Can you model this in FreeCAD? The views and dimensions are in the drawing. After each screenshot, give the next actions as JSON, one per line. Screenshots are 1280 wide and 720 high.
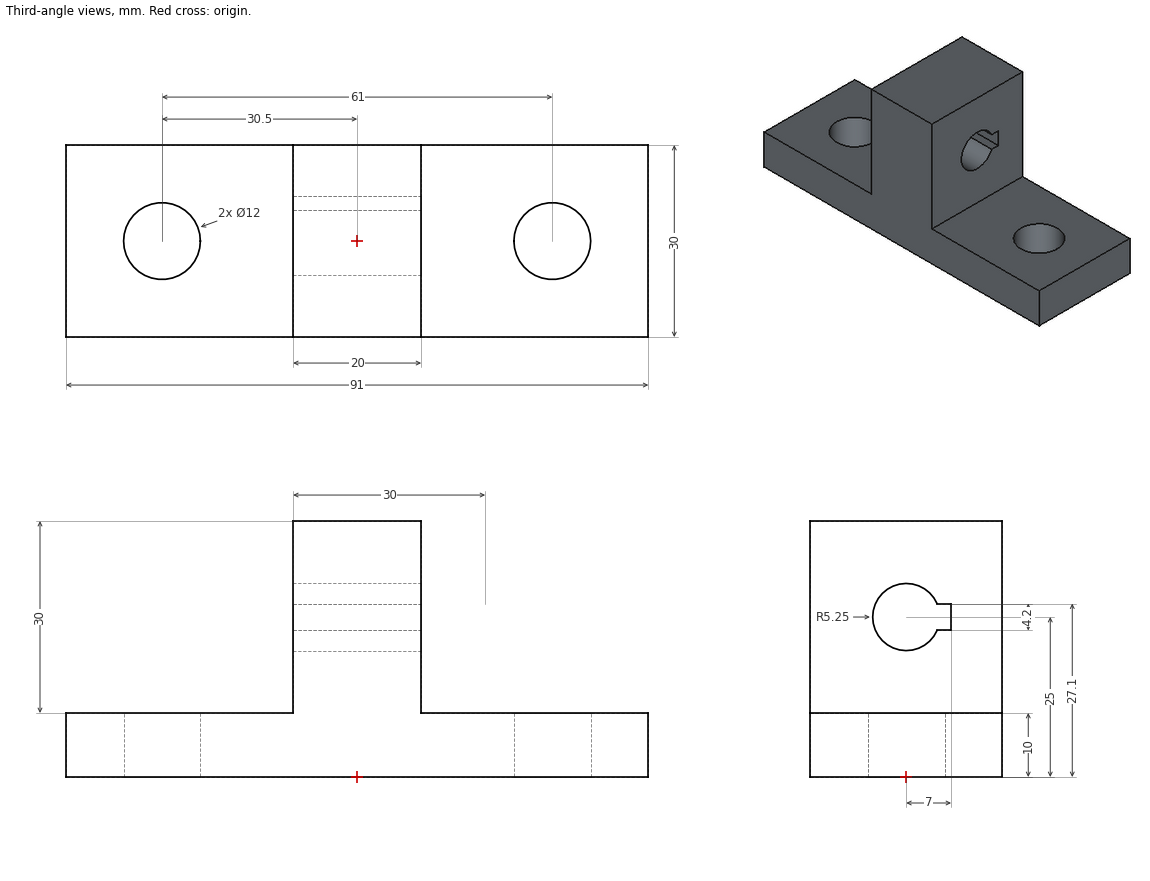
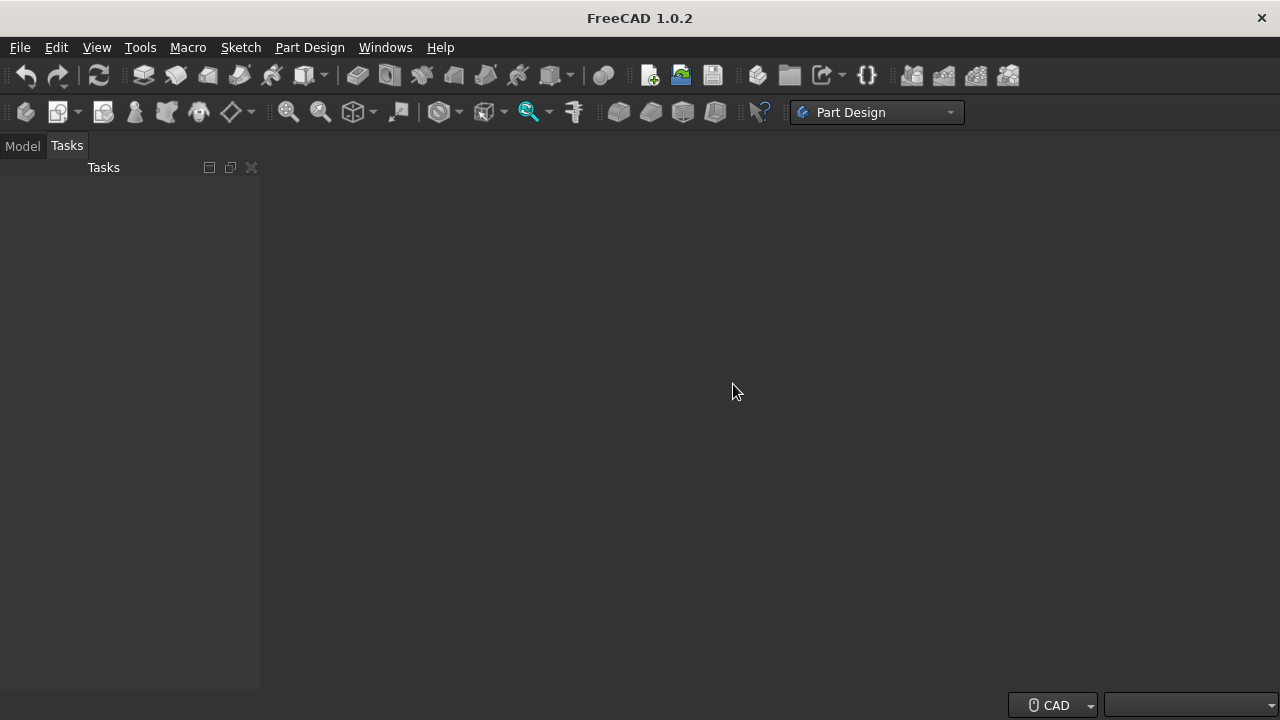
{"action": "key", "text": "ctrl+n"}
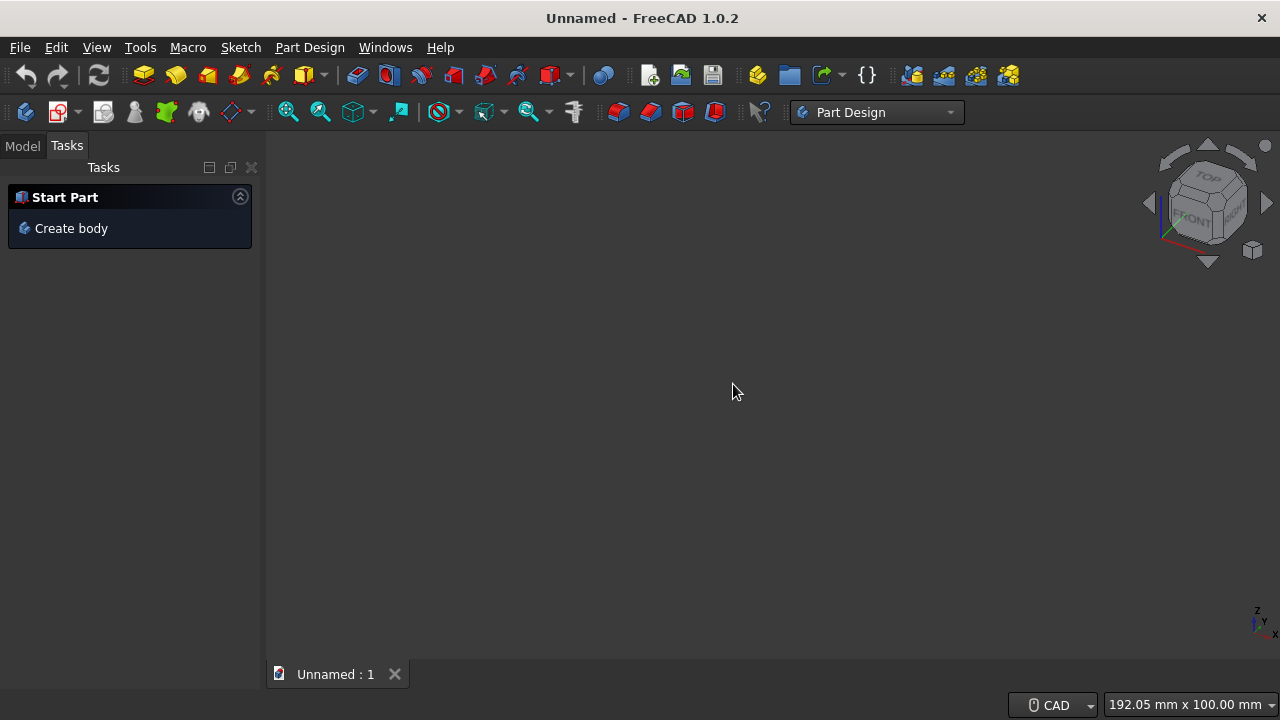
{"action": "left_click", "coordinate": [58, 112]}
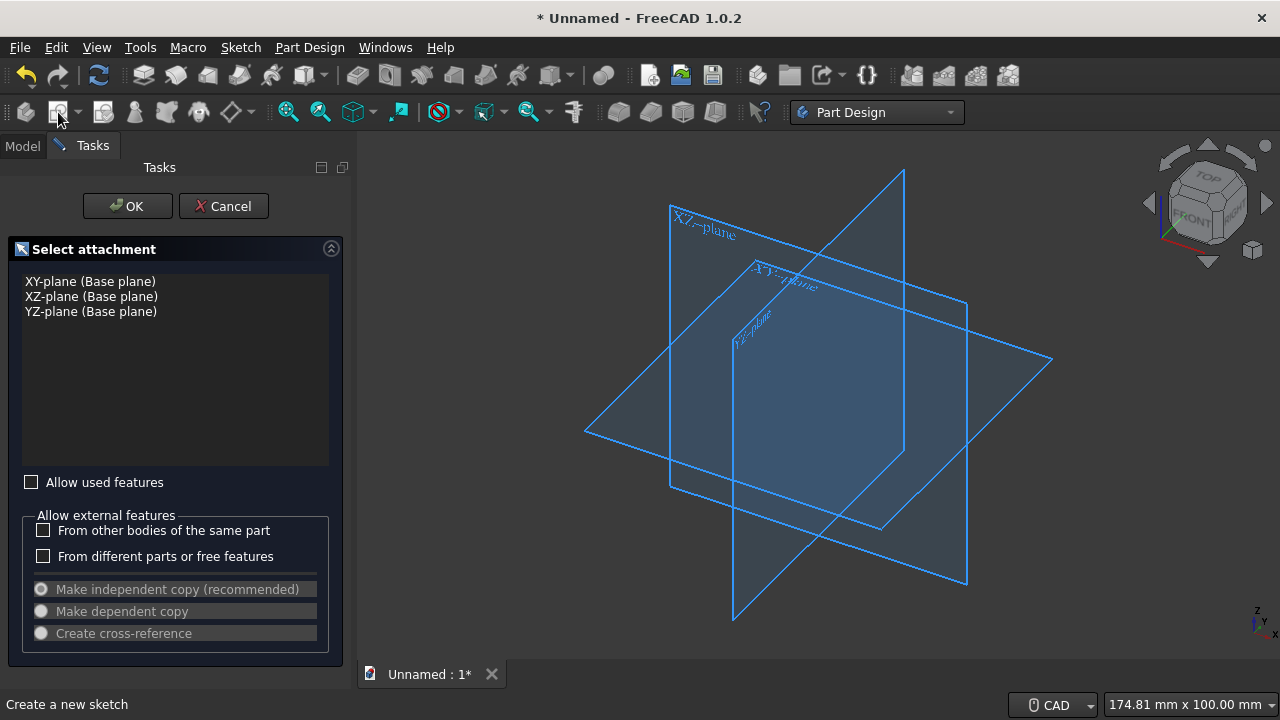
{"action": "left_click", "coordinate": [82, 282]}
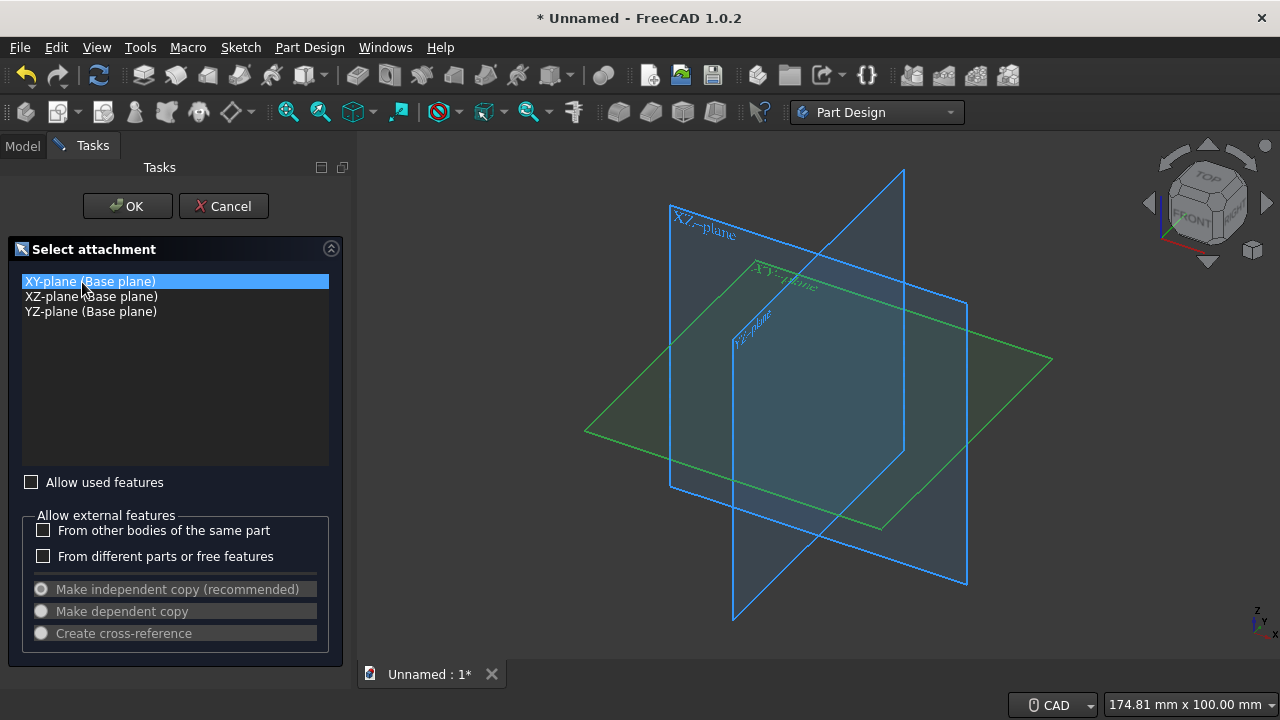
{"action": "left_click", "coordinate": [128, 206]}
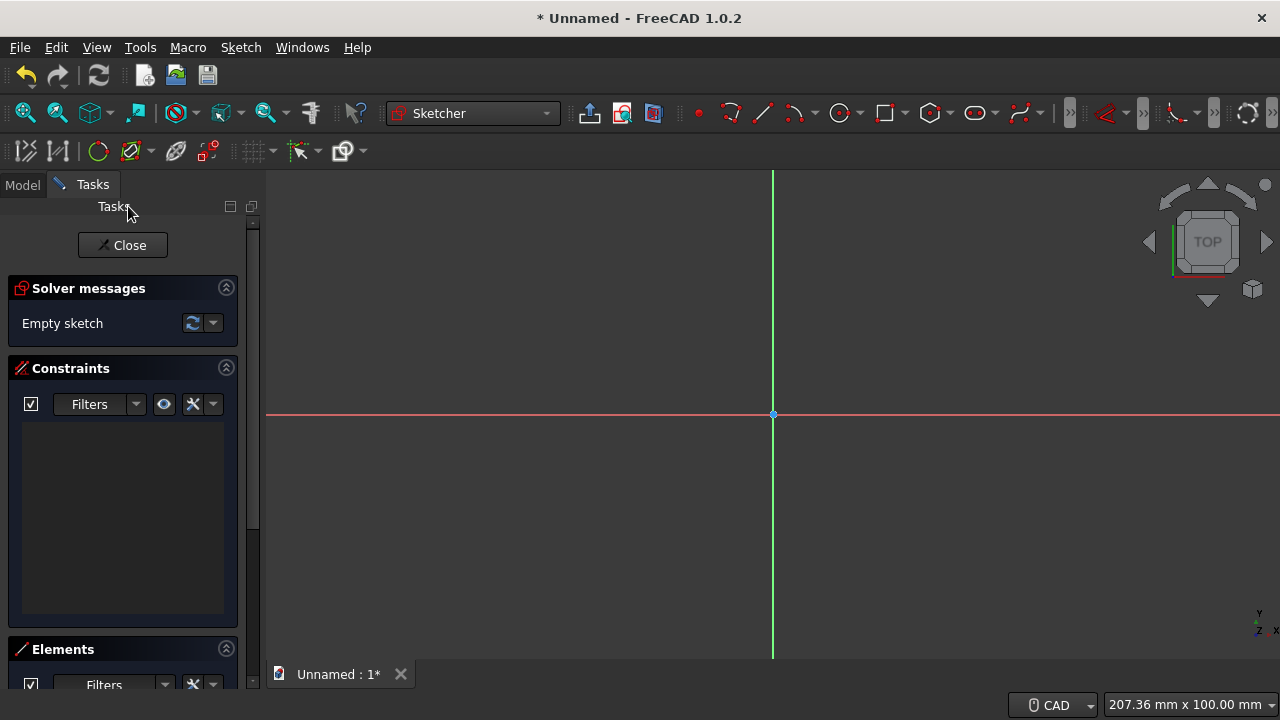
{"action": "key", "text": "g v"}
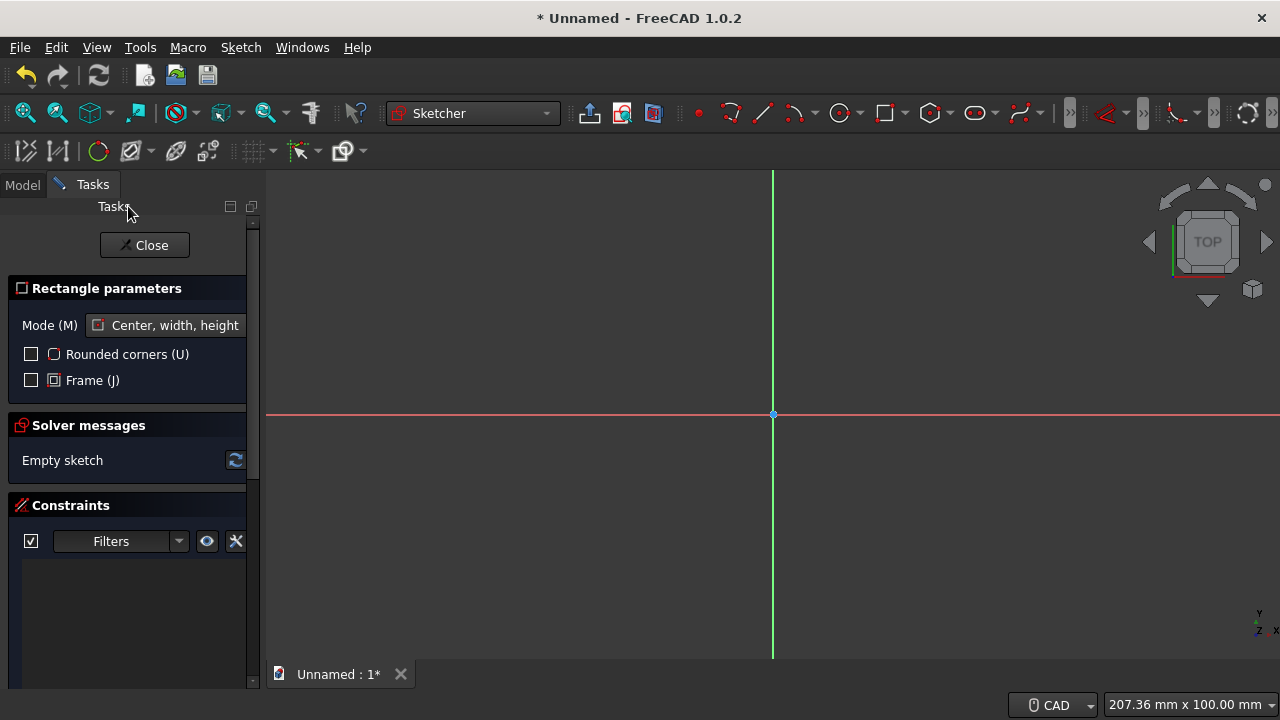
{"action": "left_click", "coordinate": [773, 414]}
{"action": "left_click", "coordinate": [995, 341]}
{"action": "key", "text": "Escape"}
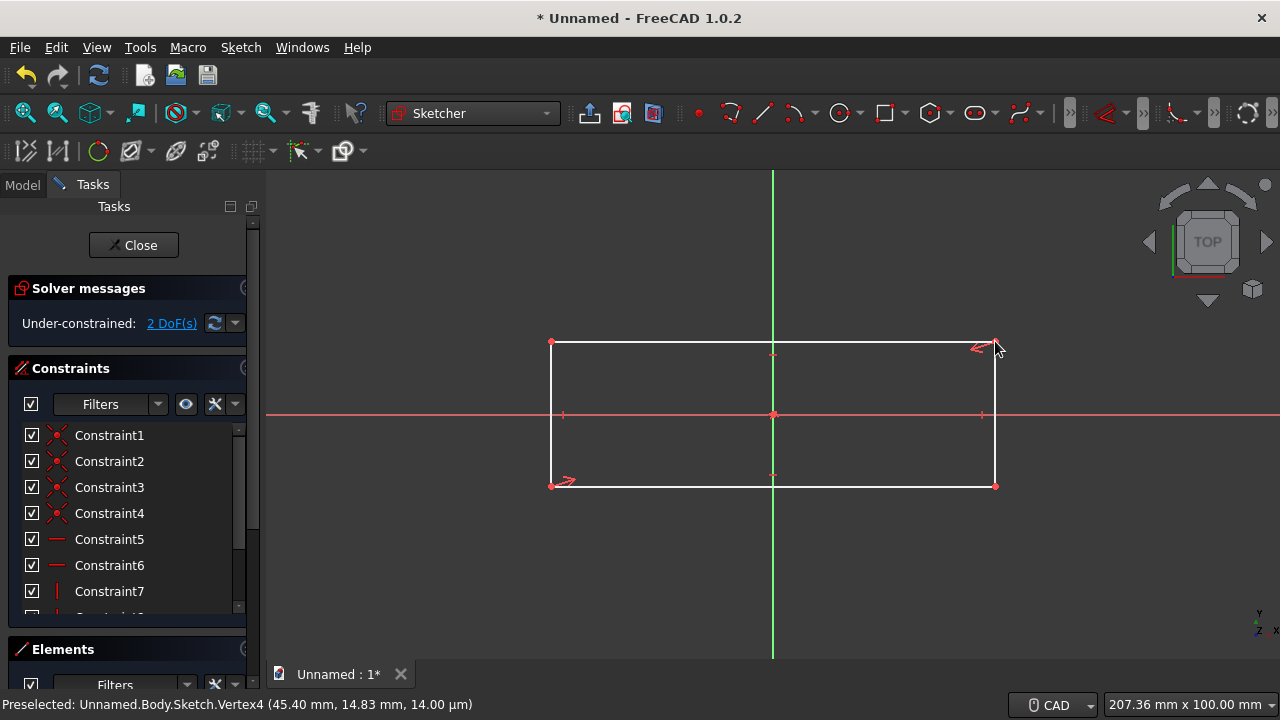
{"action": "key", "text": "d"}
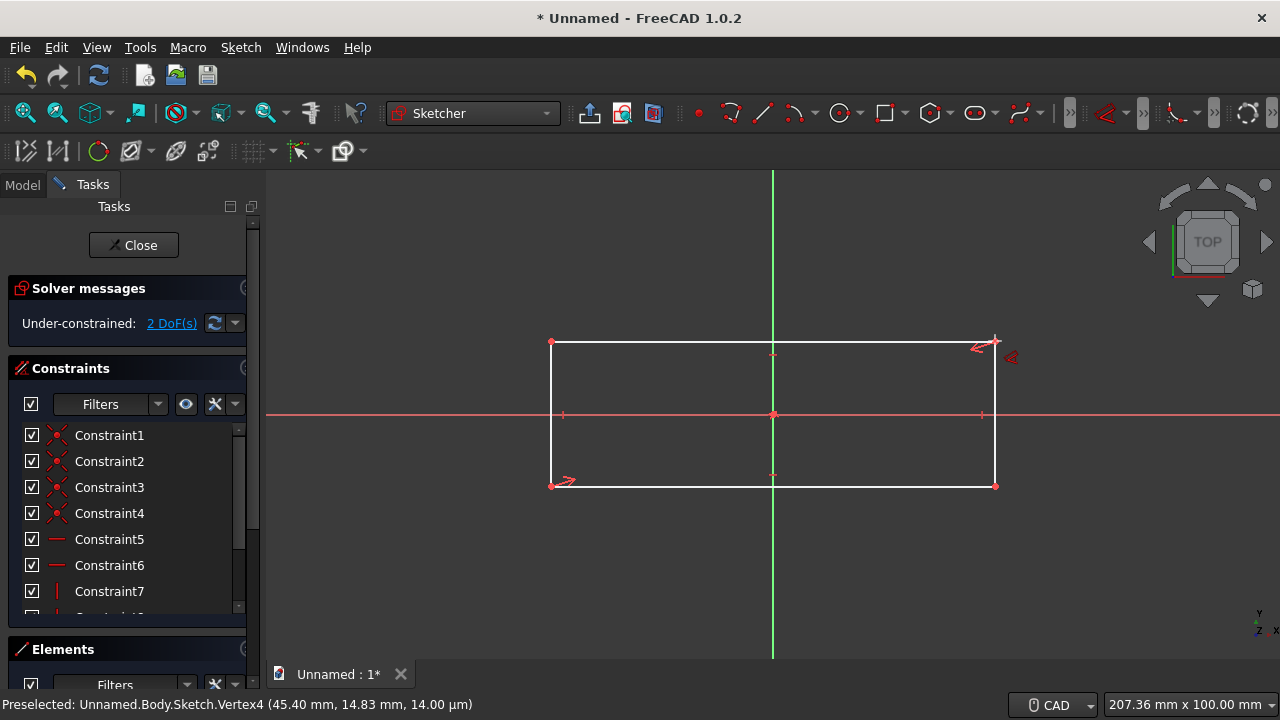
{"action": "left_click", "coordinate": [684, 487]}
{"action": "left_click", "coordinate": [671, 521]}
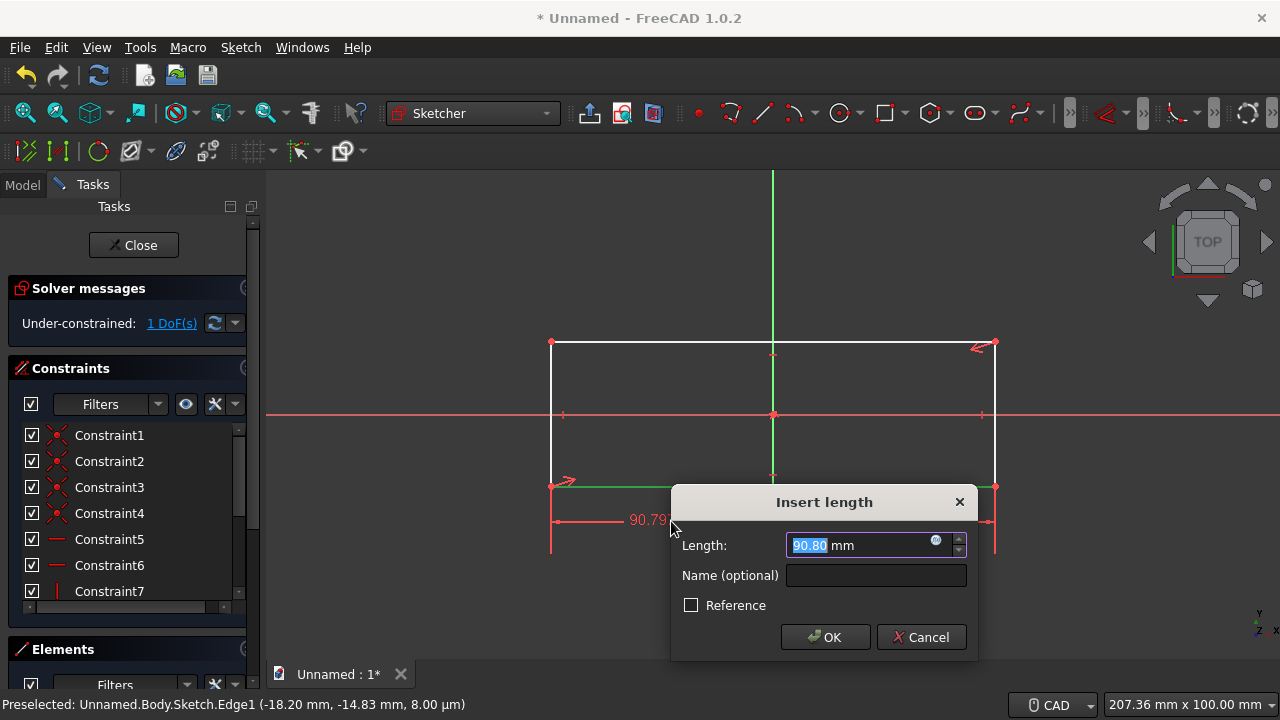
{"action": "type", "text": "91"}
{"action": "key", "text": "Return"}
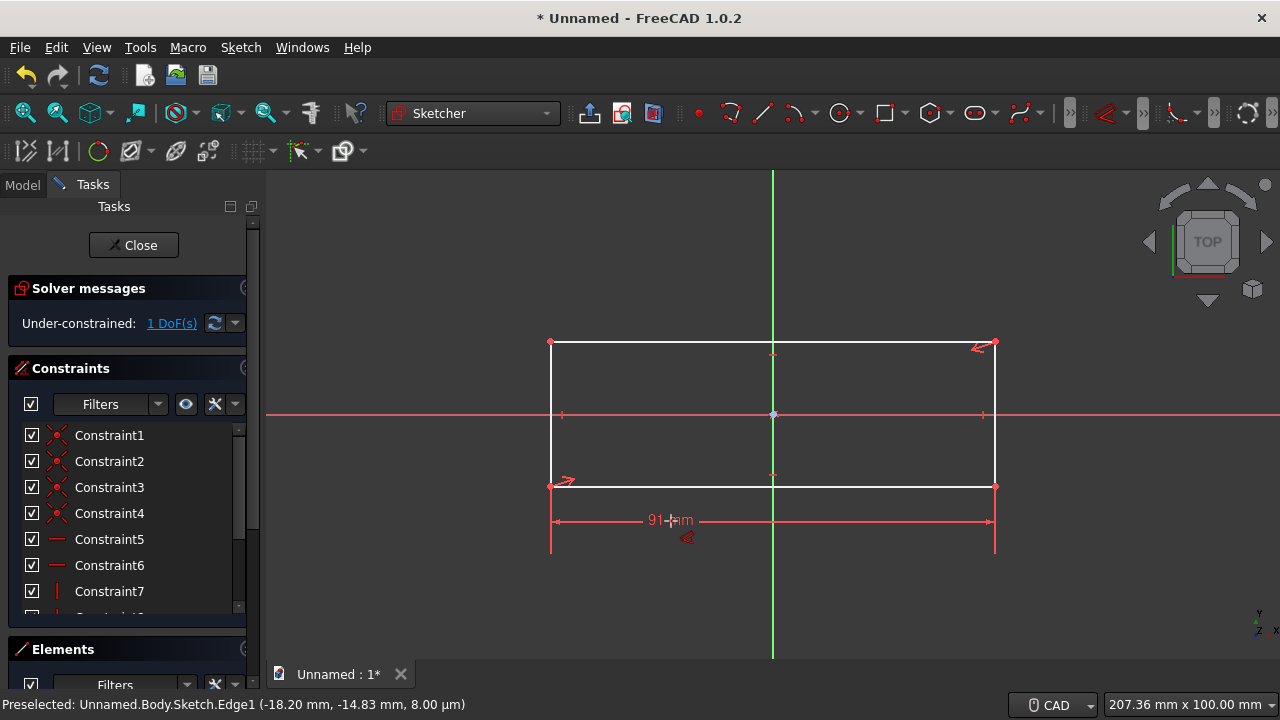
{"action": "left_click", "coordinate": [995, 444]}
{"action": "left_click", "coordinate": [1029, 381]}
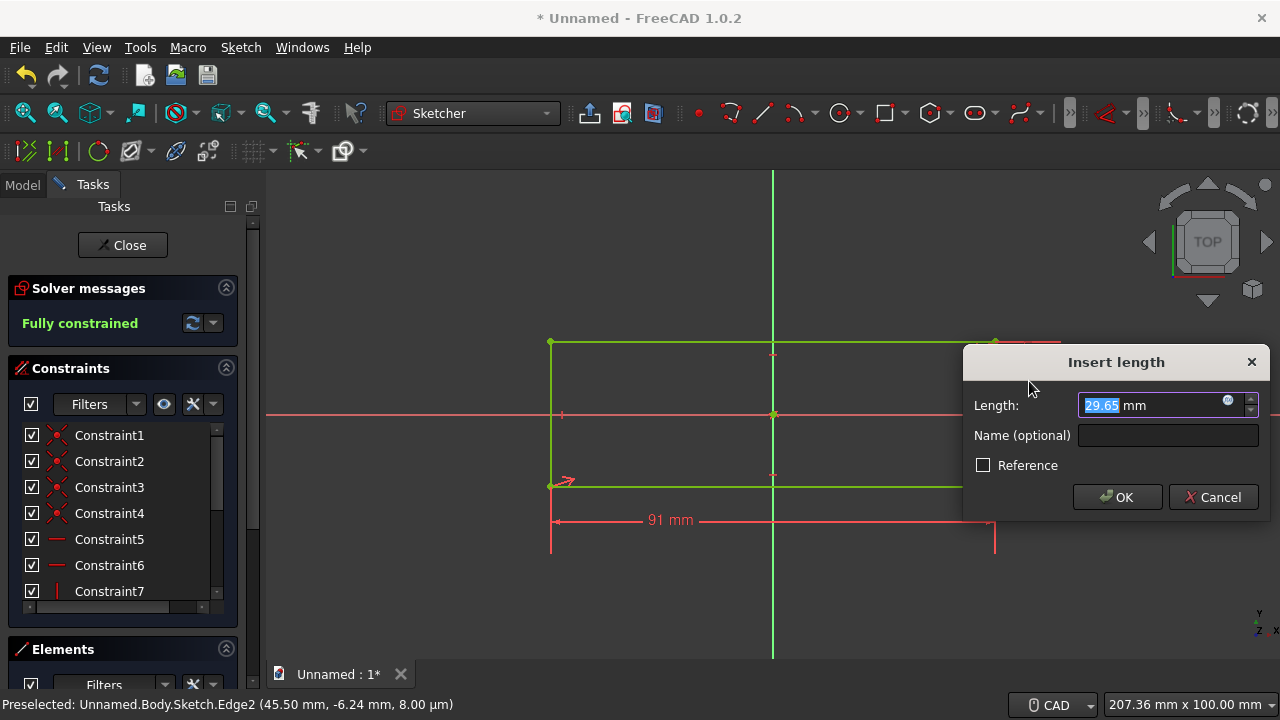
{"action": "type", "text": "30"}
{"action": "key", "text": "Return"}
{"action": "key", "text": "Escape"}